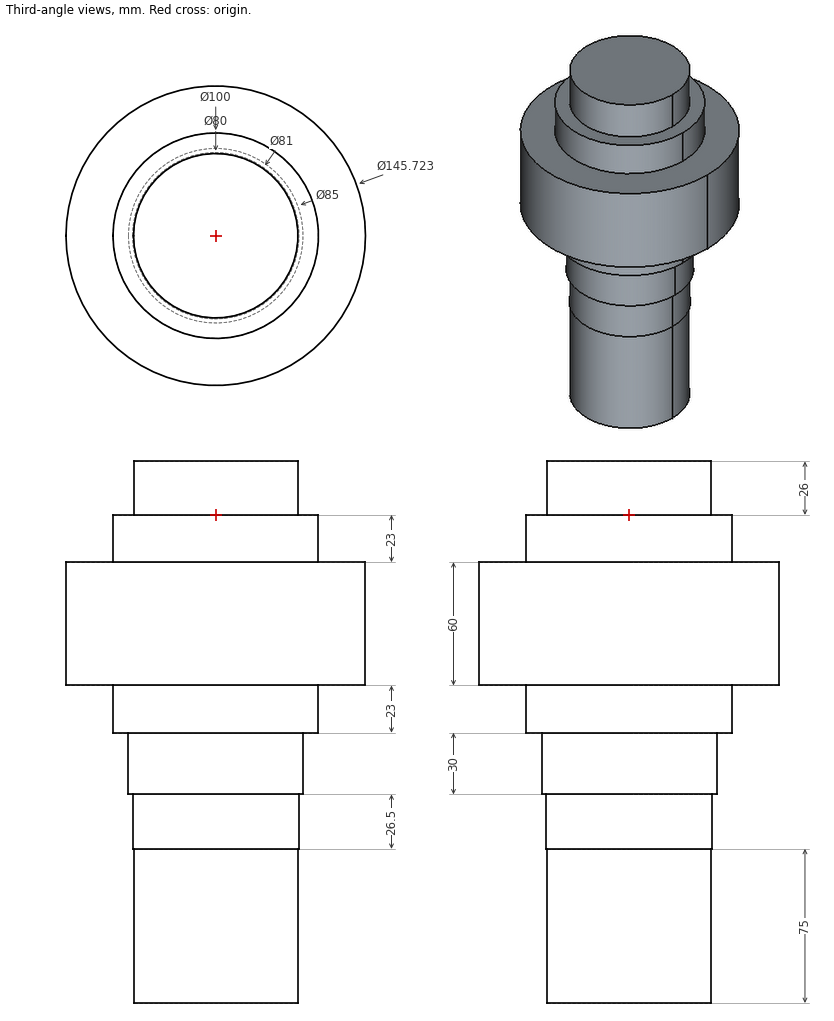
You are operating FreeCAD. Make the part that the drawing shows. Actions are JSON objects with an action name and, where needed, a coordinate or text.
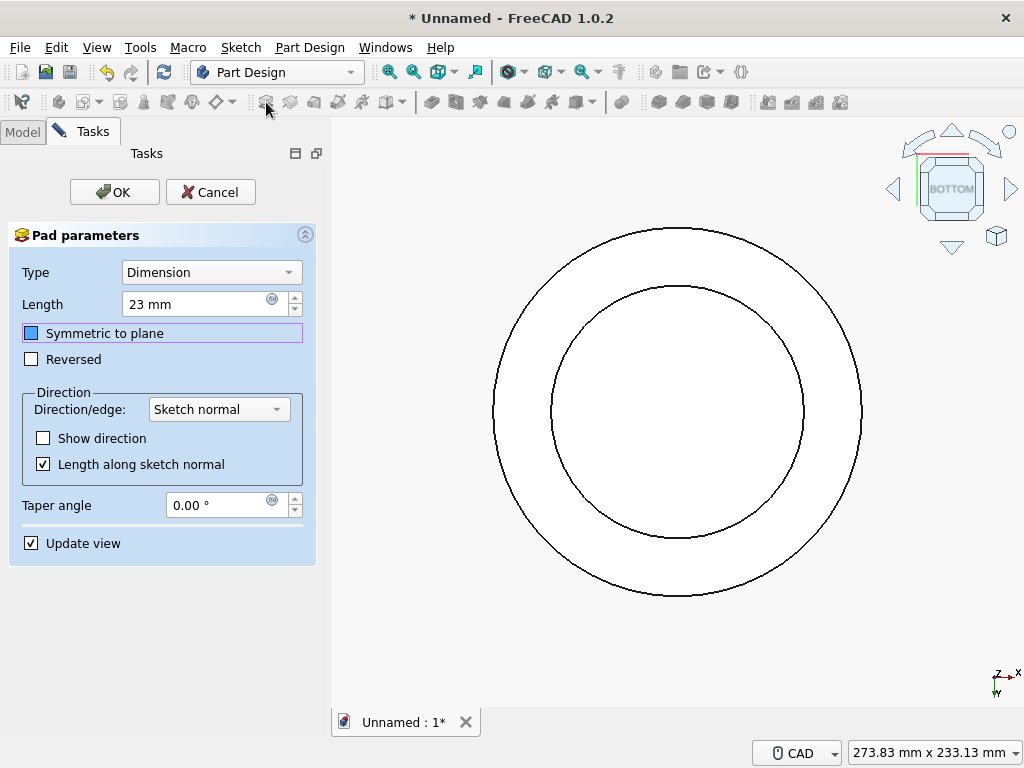
{"action": "left_click", "coordinate": [115, 192]}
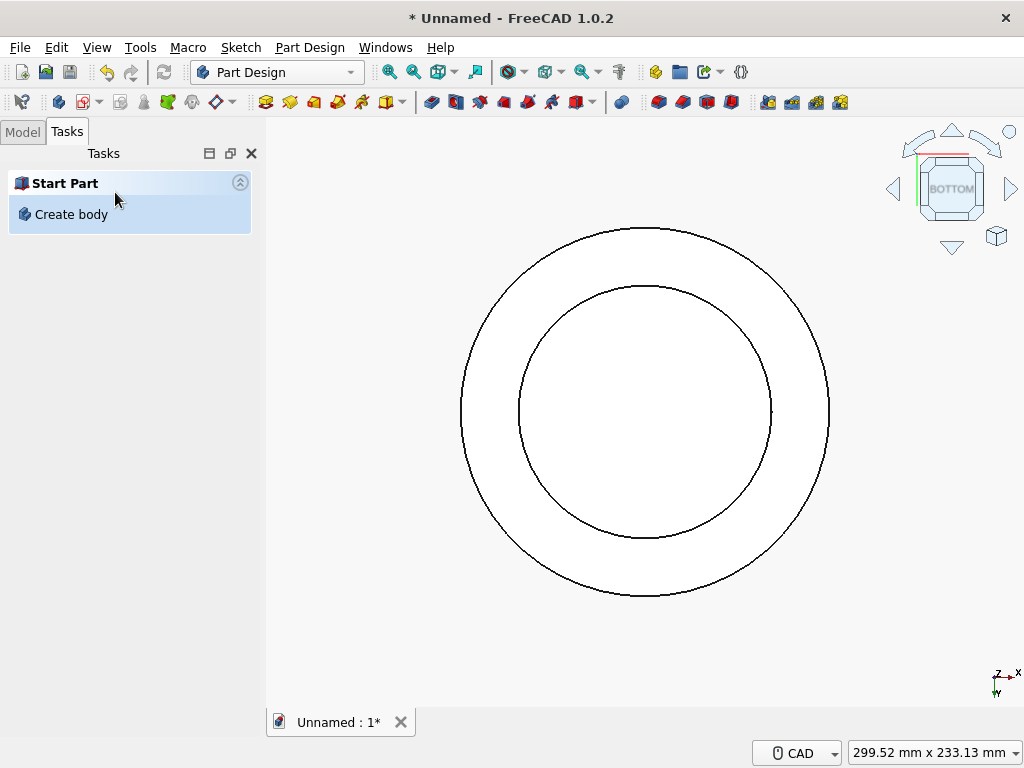
{"action": "left_click", "coordinate": [645, 411]}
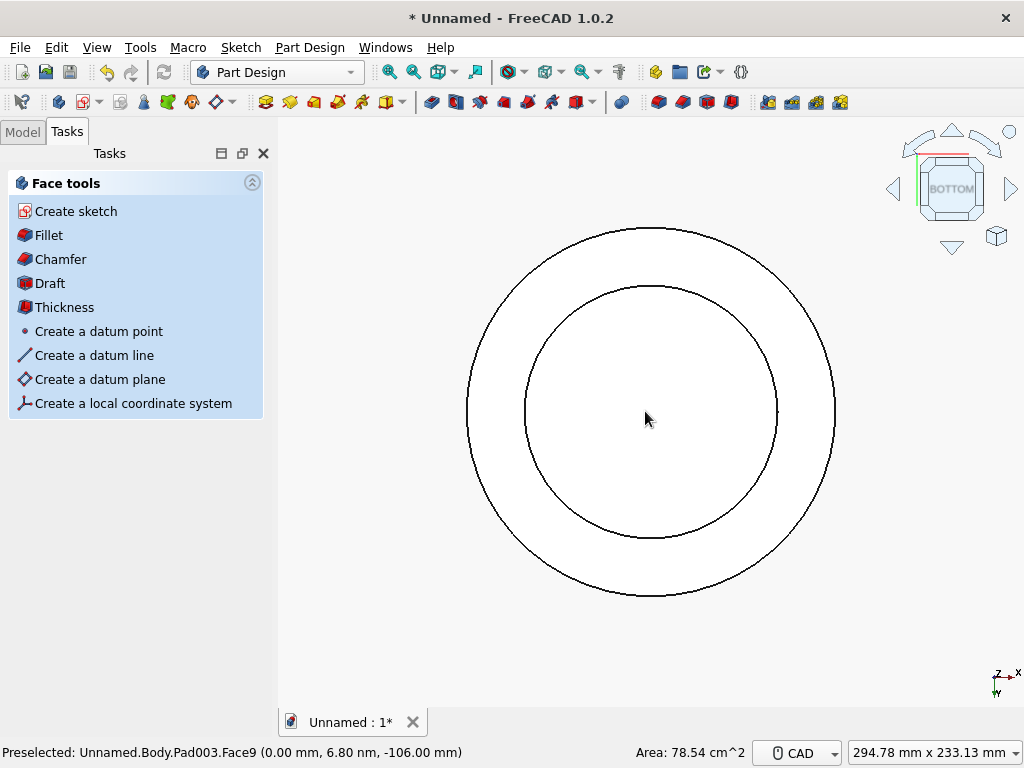
{"action": "left_click", "coordinate": [84, 102]}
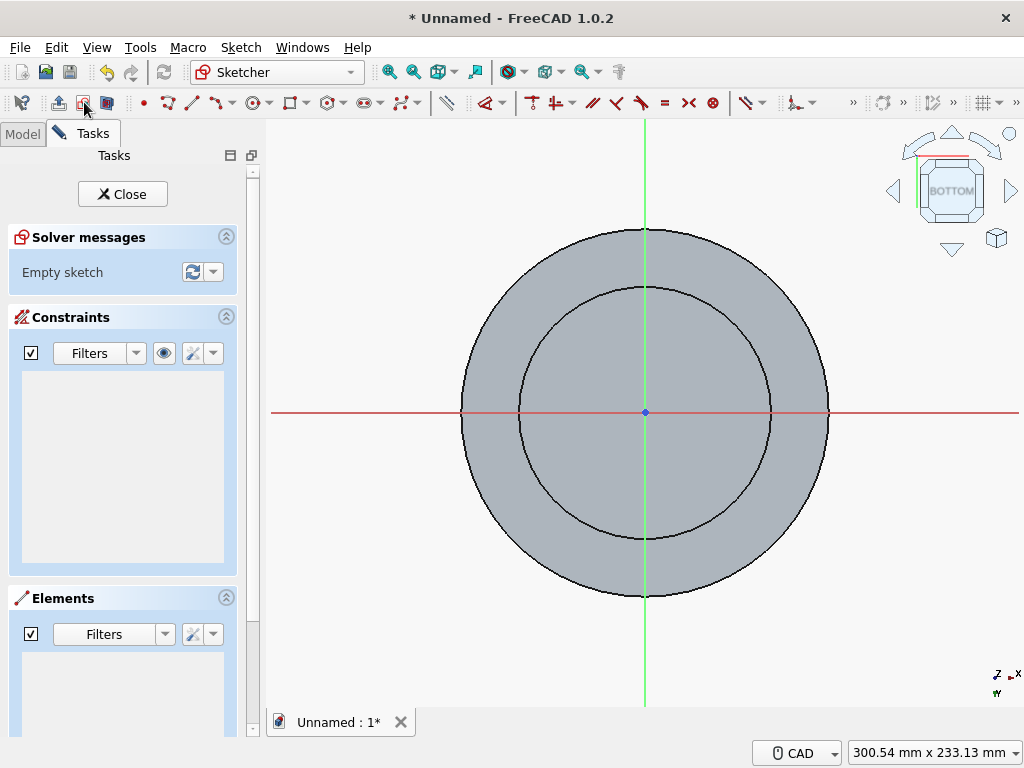
{"action": "scroll", "coordinate": [728, 413], "scroll_direction": "up", "scroll_amount": 3}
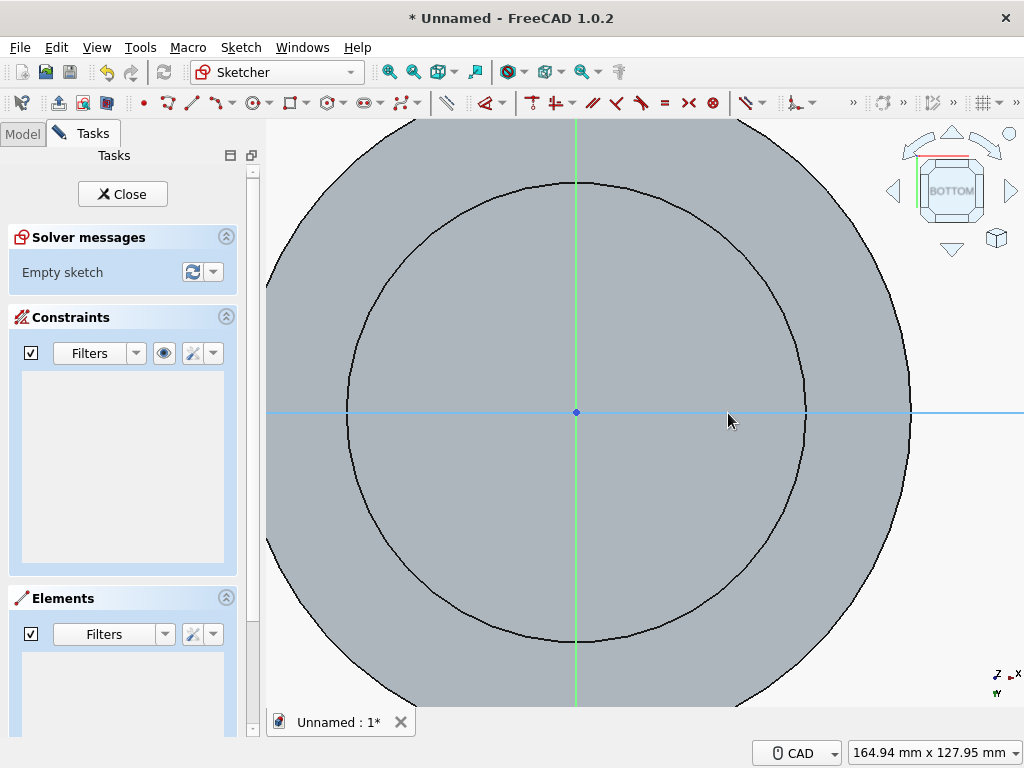
{"action": "key", "text": "g c"}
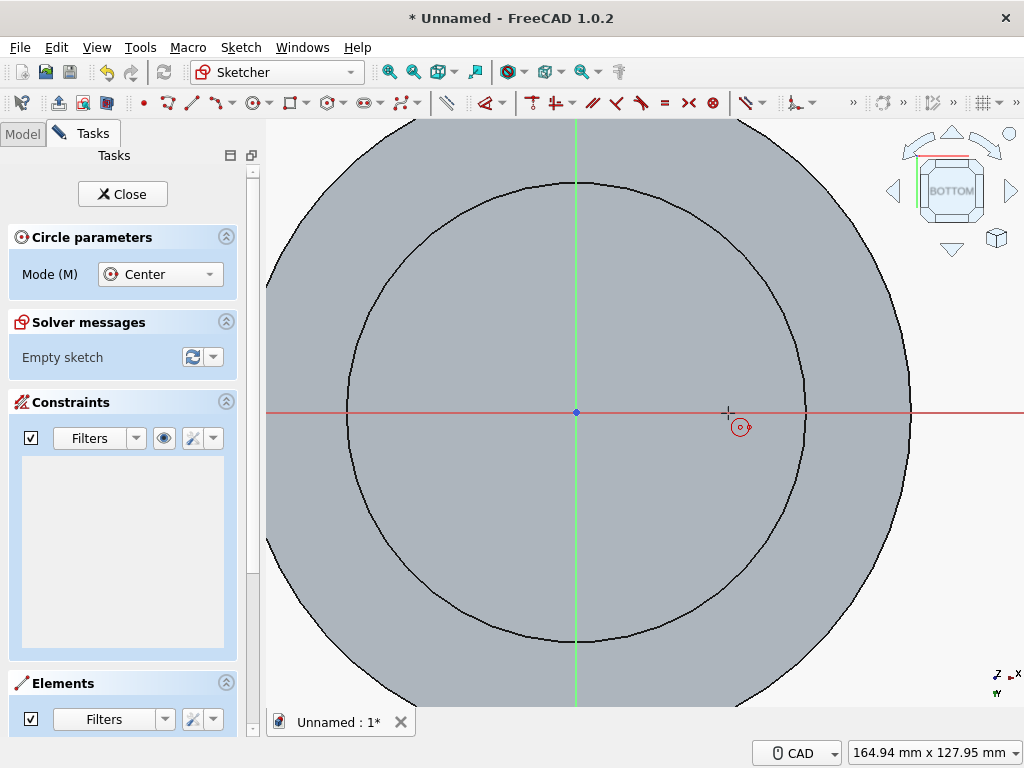
{"action": "left_click", "coordinate": [576, 413]}
{"action": "left_click", "coordinate": [714, 274]}
{"action": "key", "text": "Escape"}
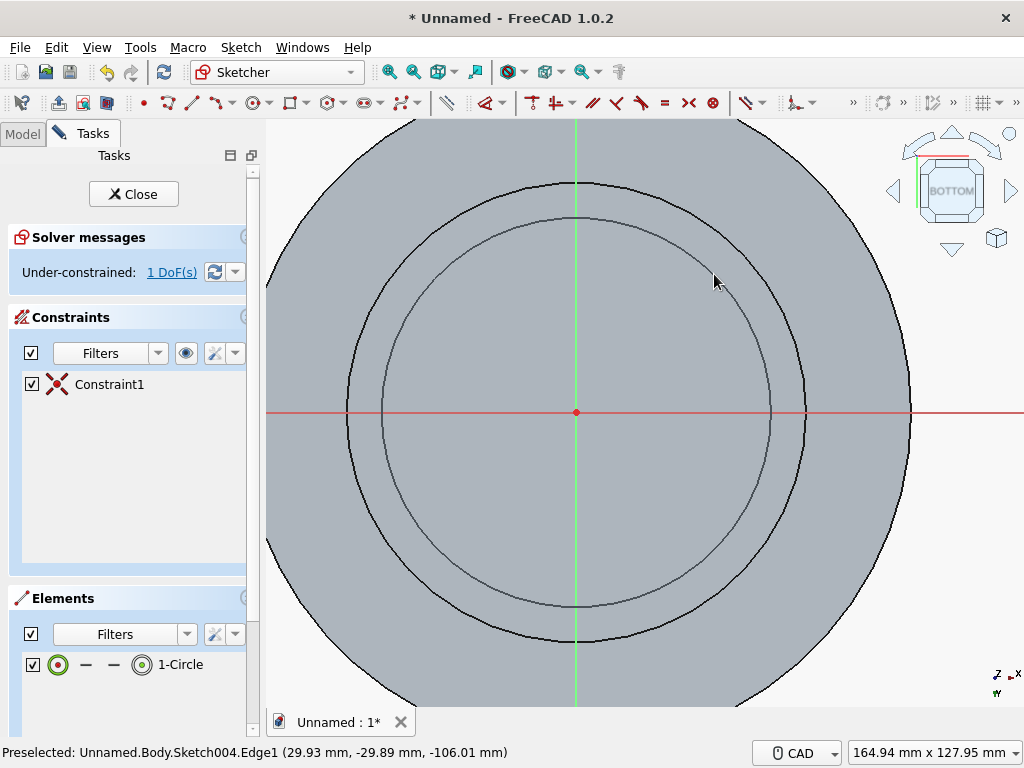
{"action": "left_click", "coordinate": [486, 104]}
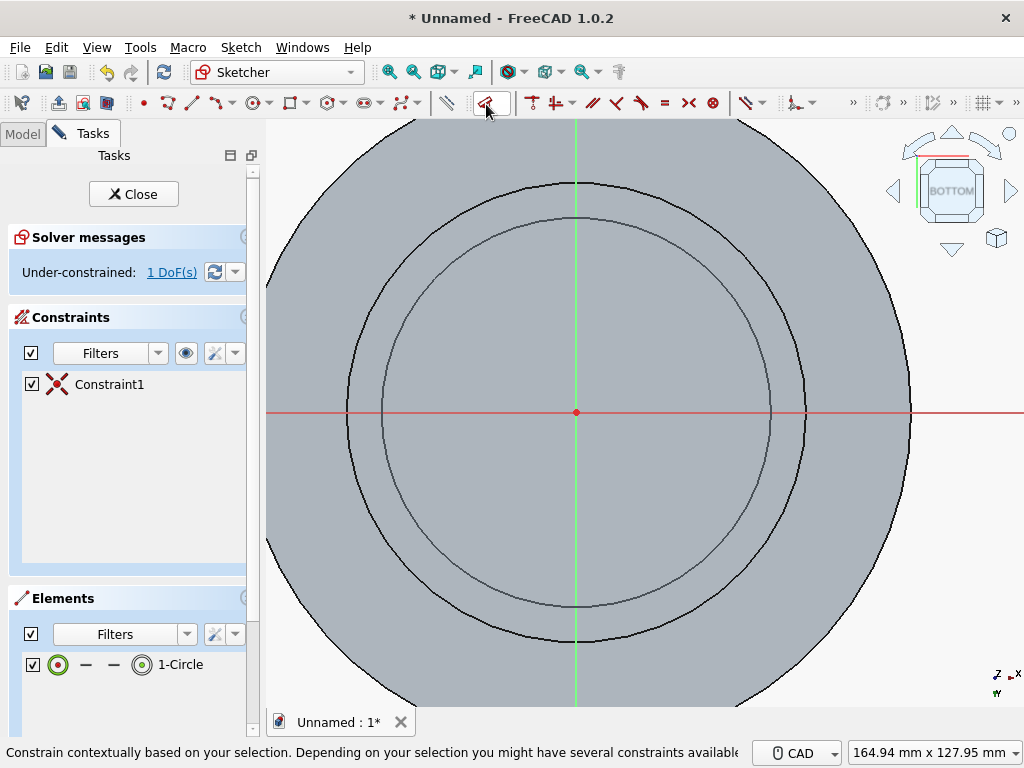
{"action": "left_click", "coordinate": [713, 274]}
{"action": "left_click", "coordinate": [735, 251]}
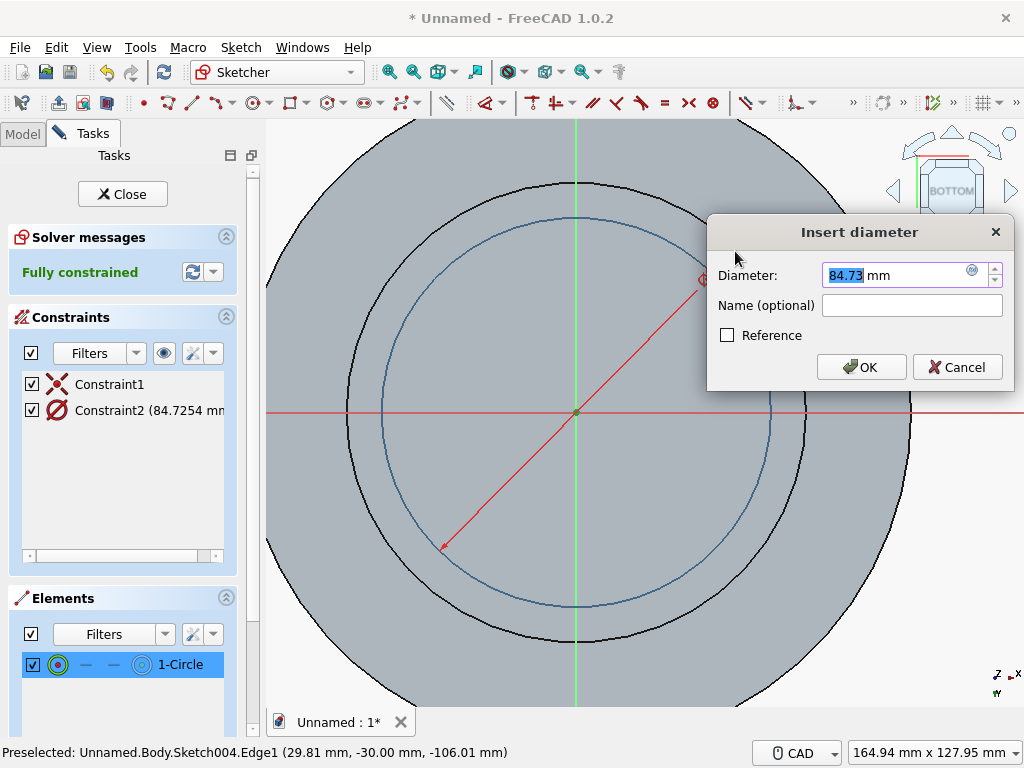
{"action": "type", "text": "85"}
{"action": "key", "text": "Return"}
{"action": "key", "text": "Escape"}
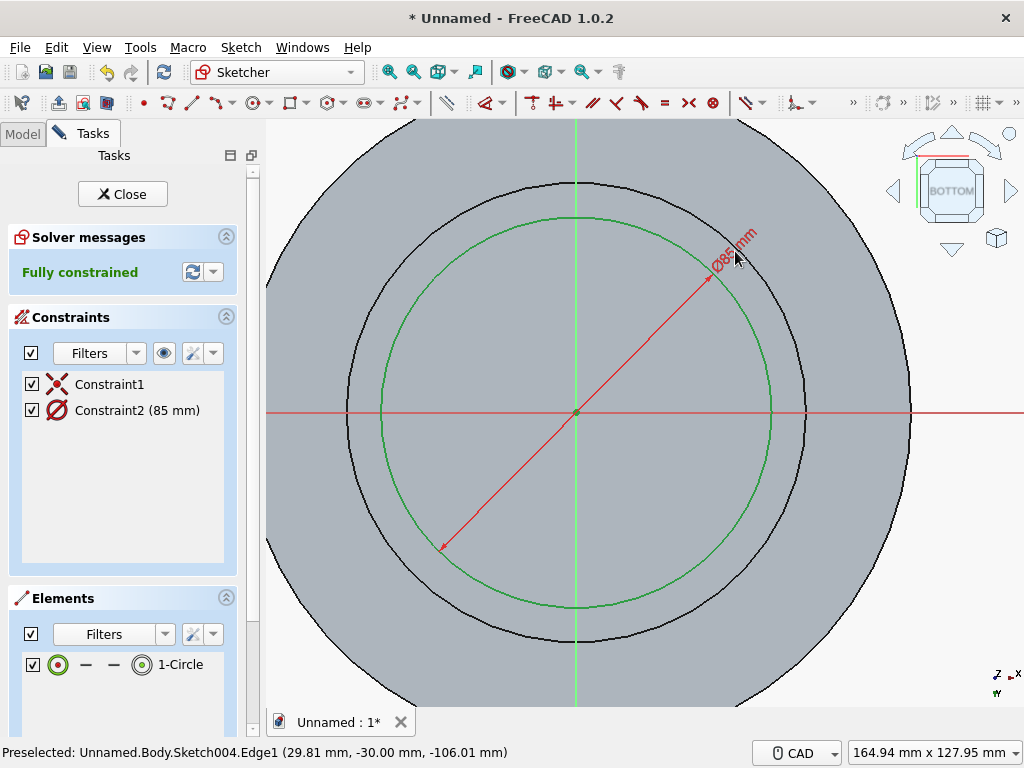
{"action": "left_click", "coordinate": [123, 194]}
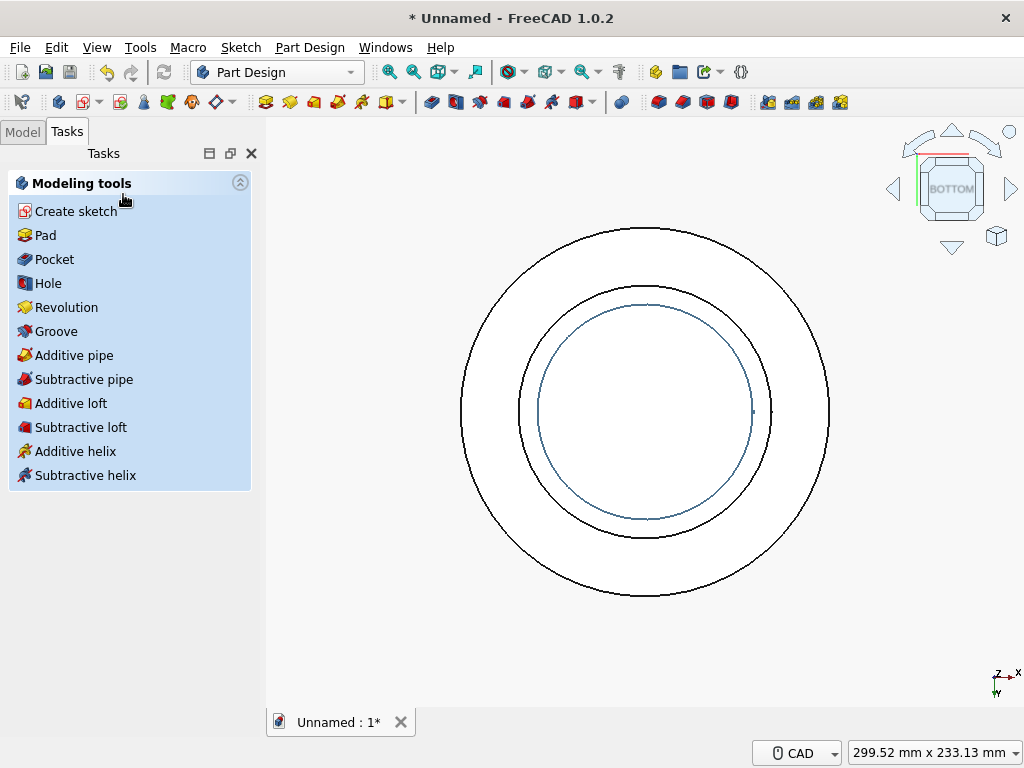
{"action": "left_click", "coordinate": [266, 102]}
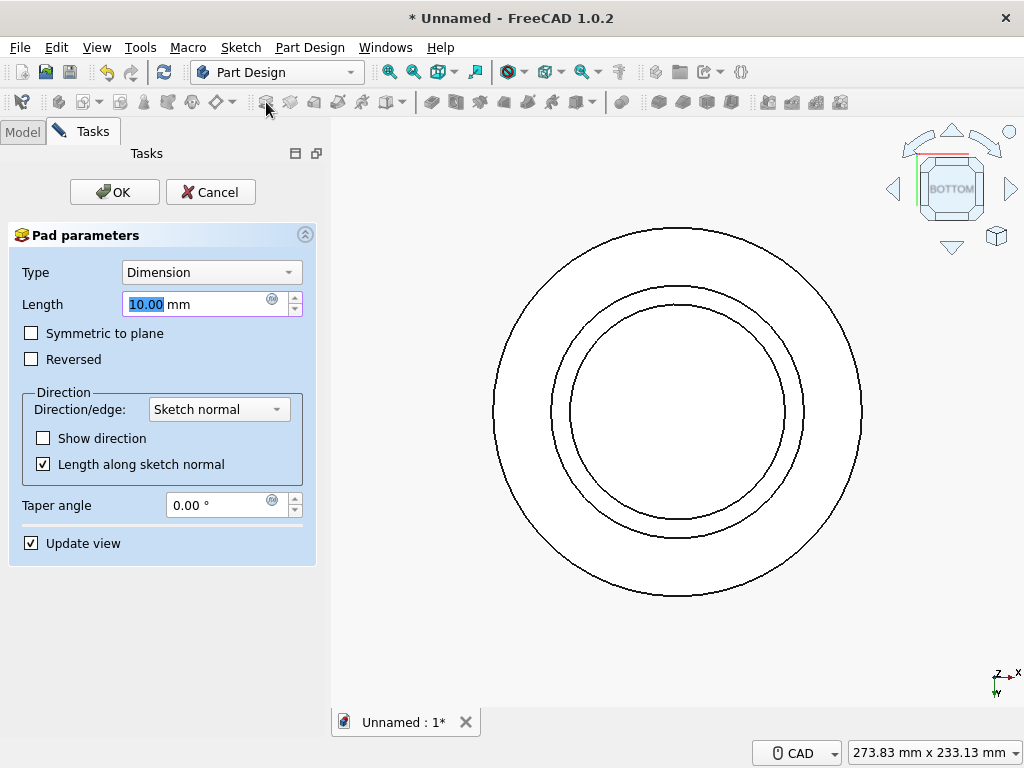
{"action": "type", "text": "30"}
{"action": "key", "text": "Tab"}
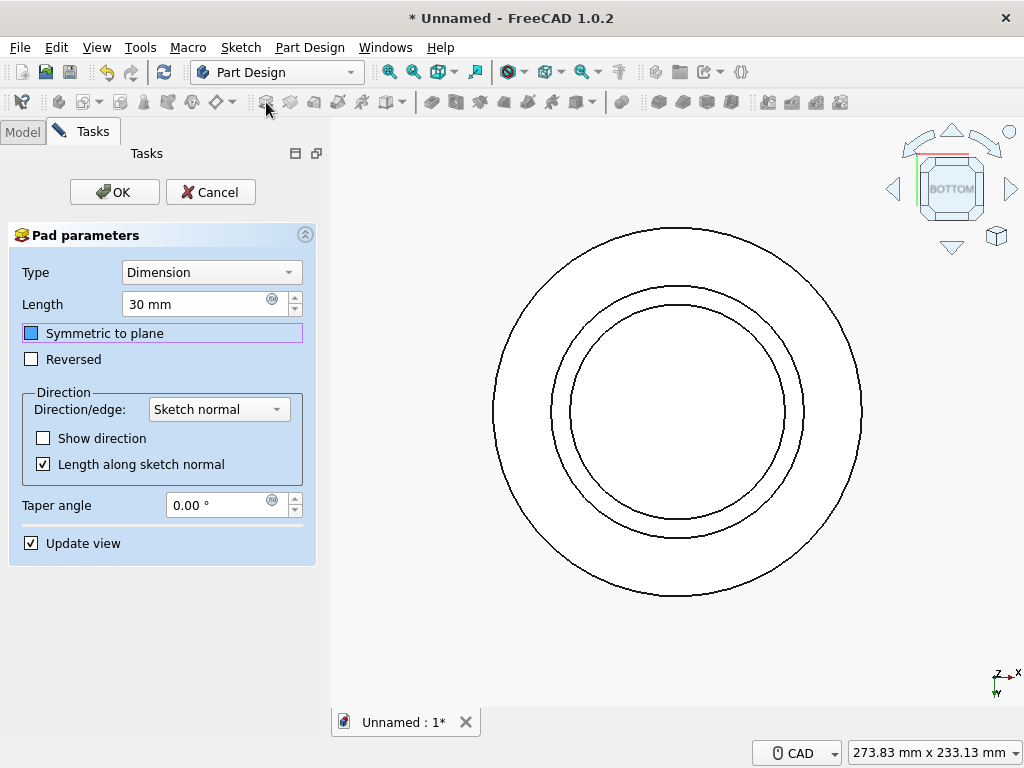
{"action": "left_click", "coordinate": [115, 192]}